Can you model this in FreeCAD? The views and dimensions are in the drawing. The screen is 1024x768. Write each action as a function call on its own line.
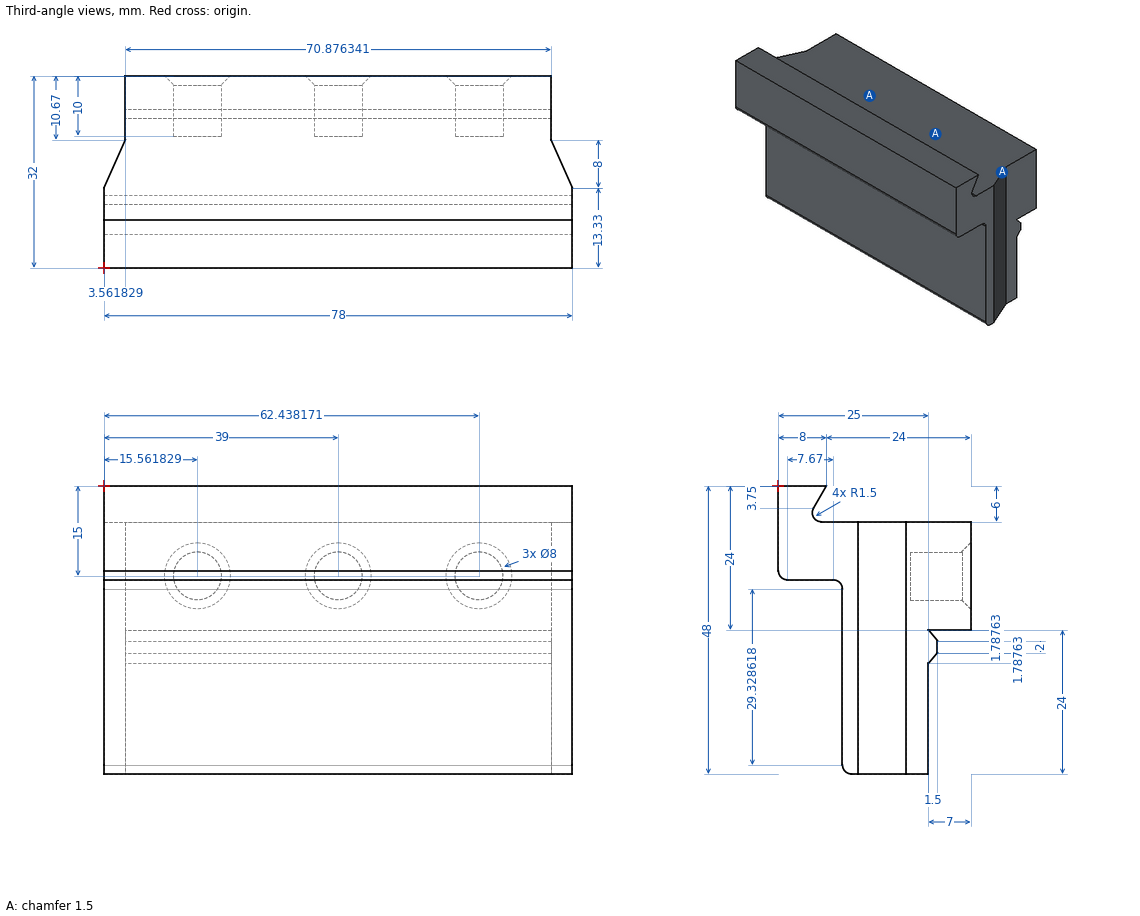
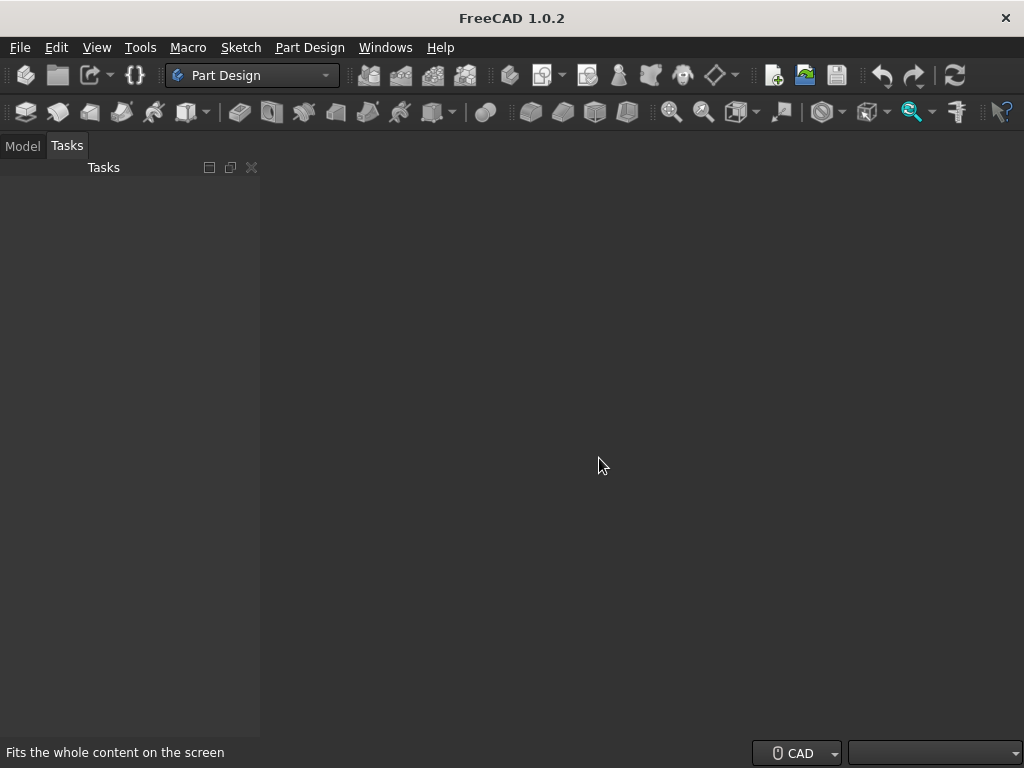
click(774, 76)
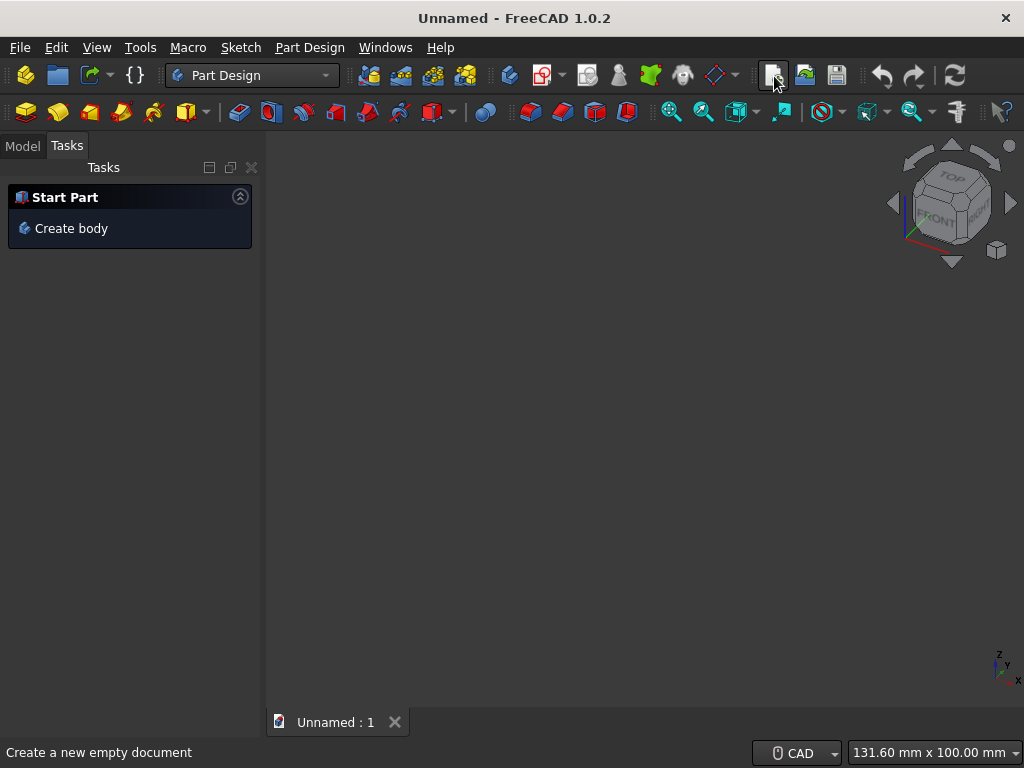
click(542, 76)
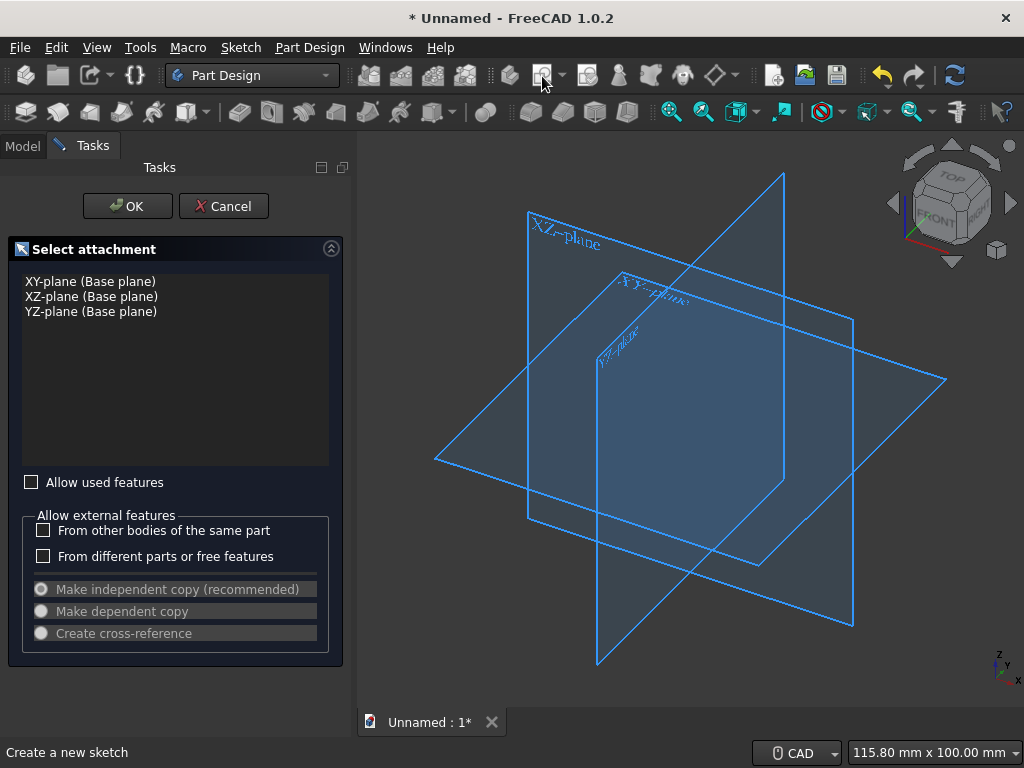
click(82, 282)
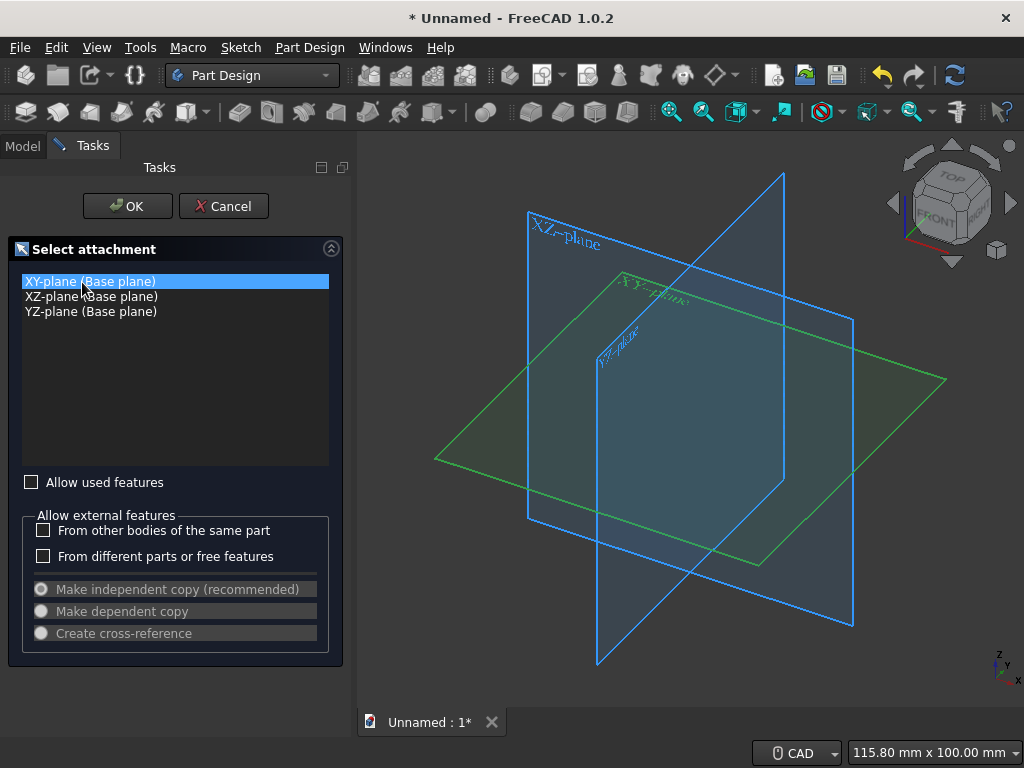
click(128, 206)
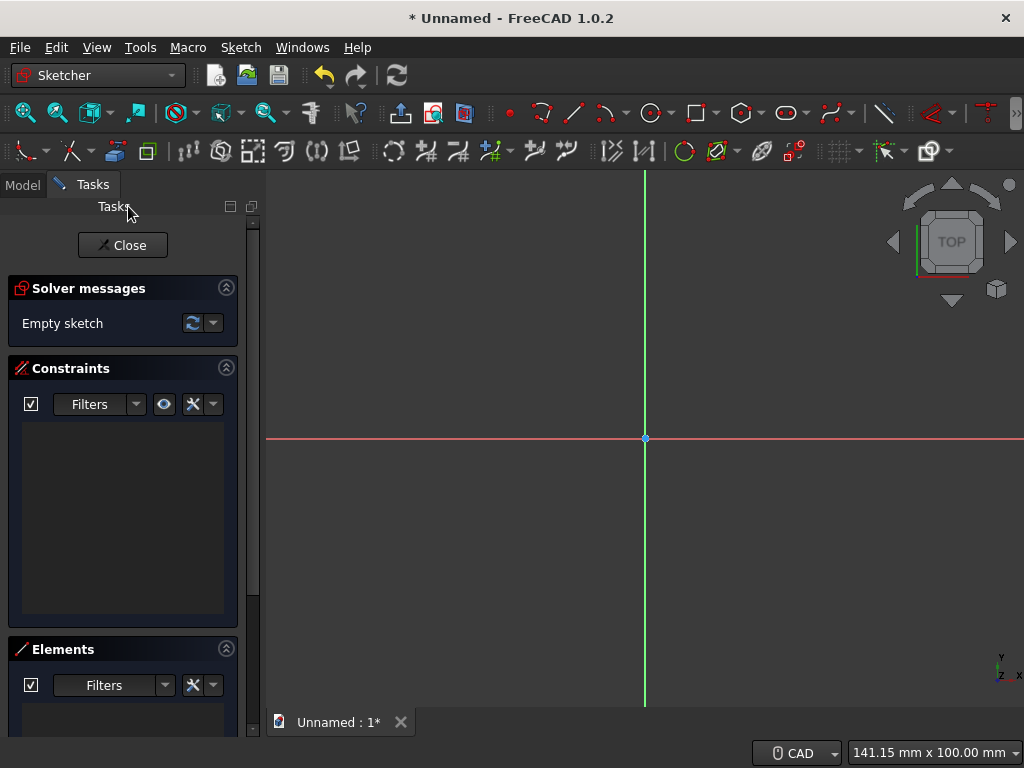
scroll(294, 613, down, 2)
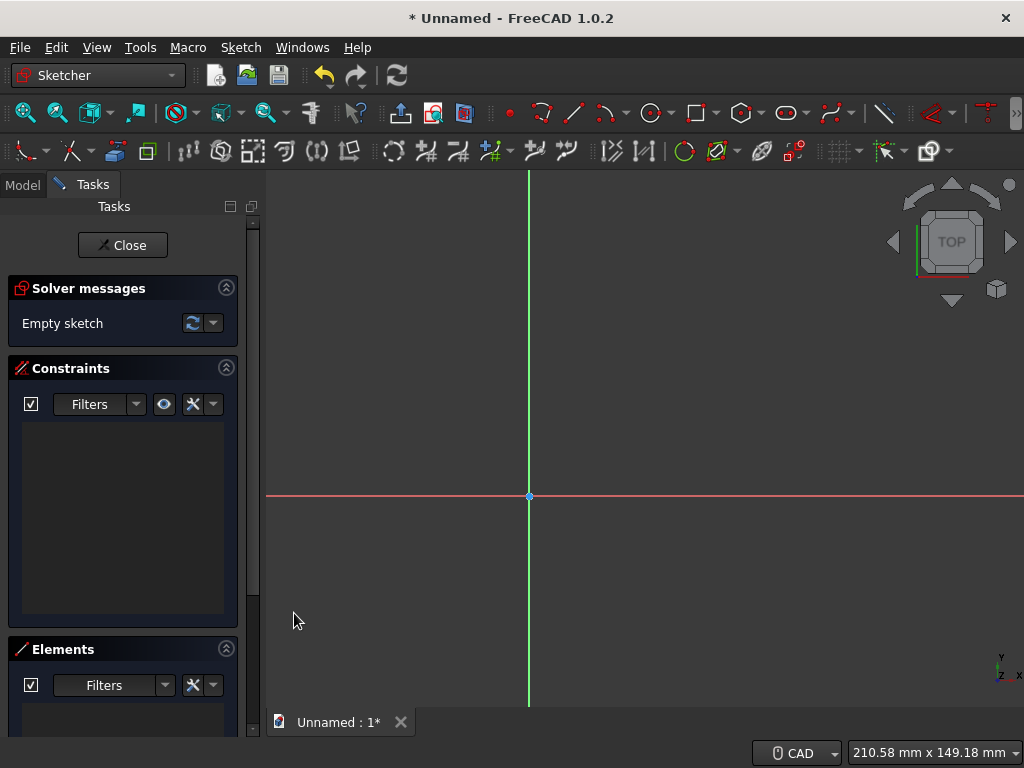
scroll(859, 439, up, 2)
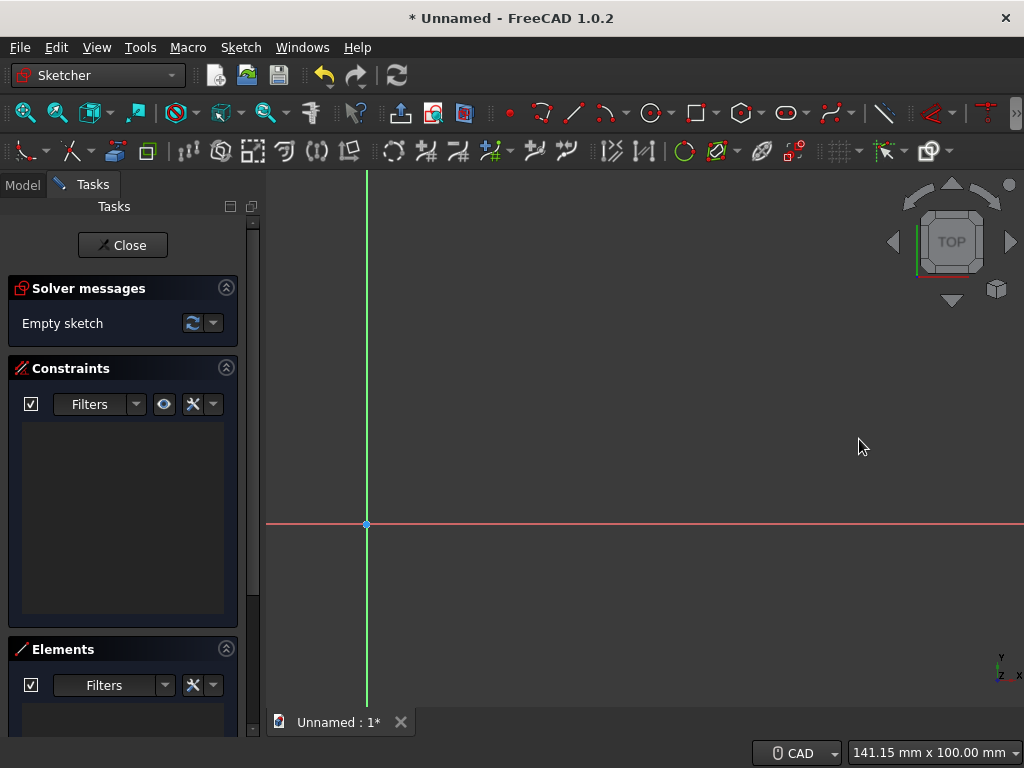
click(542, 114)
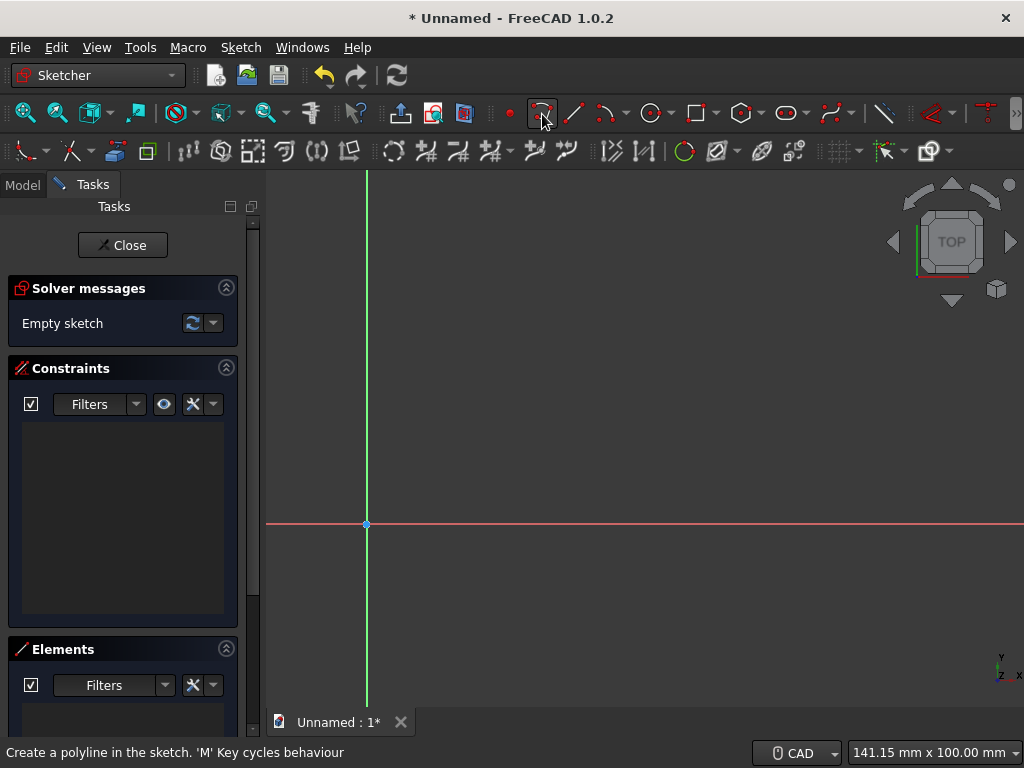
click(367, 524)
click(786, 515)
click(786, 453)
click(766, 410)
click(766, 352)
click(386, 352)
click(386, 410)
click(376, 453)
click(367, 524)
key(Escape)
key(Escape)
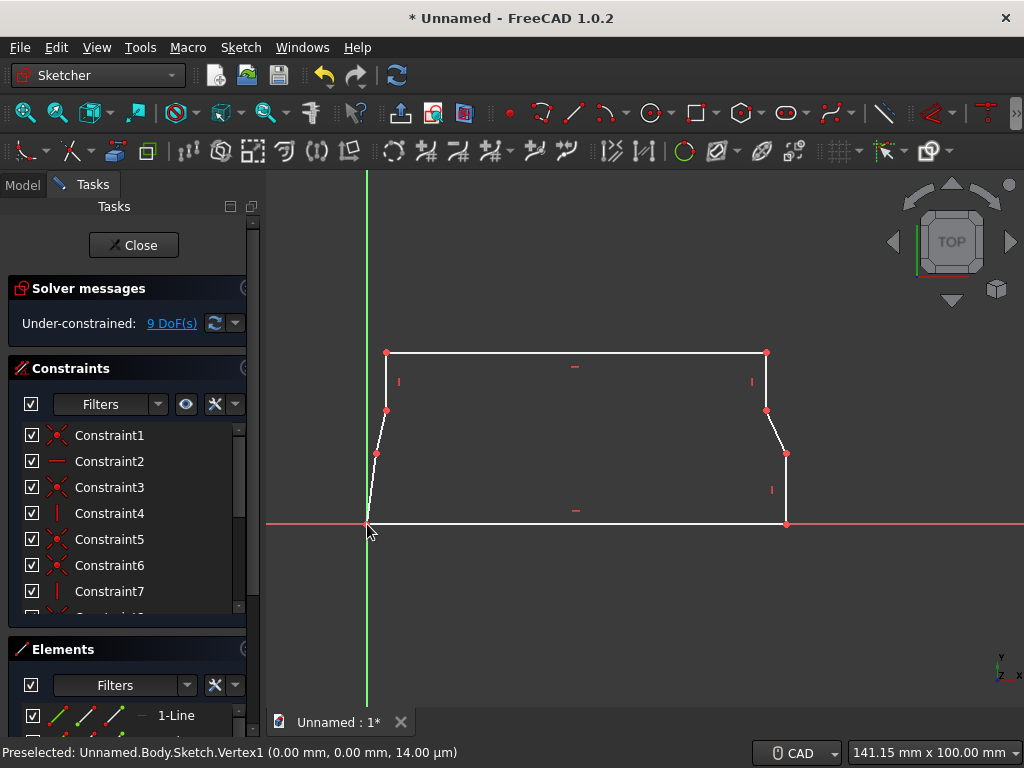
click(370, 503)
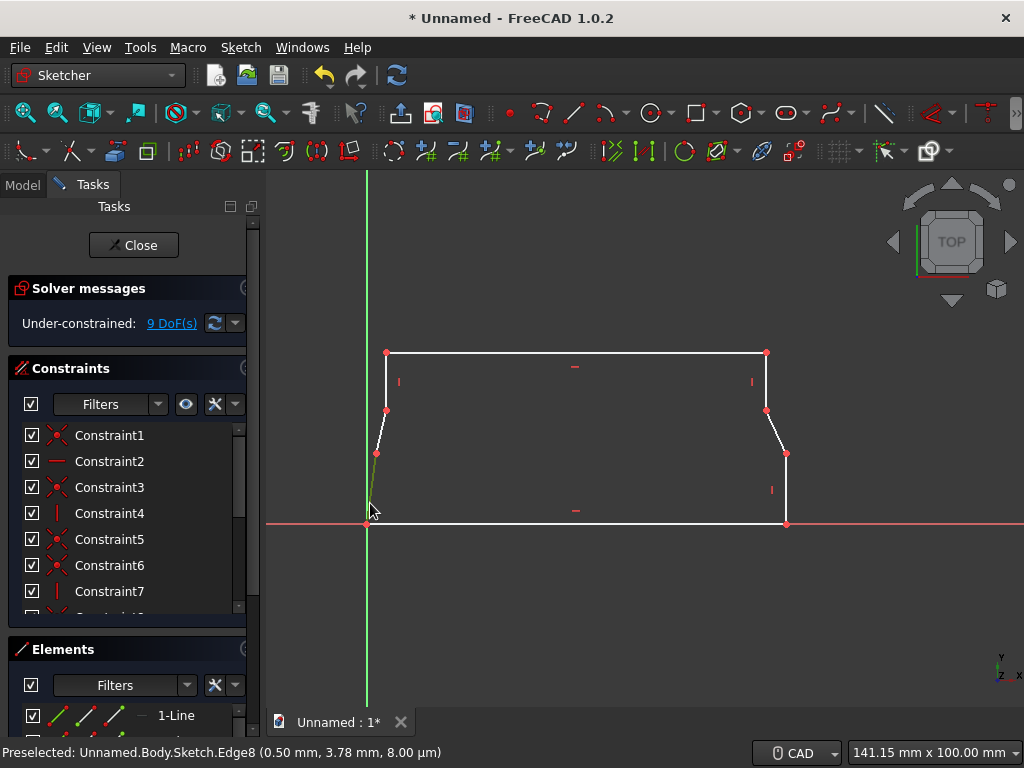
key(v)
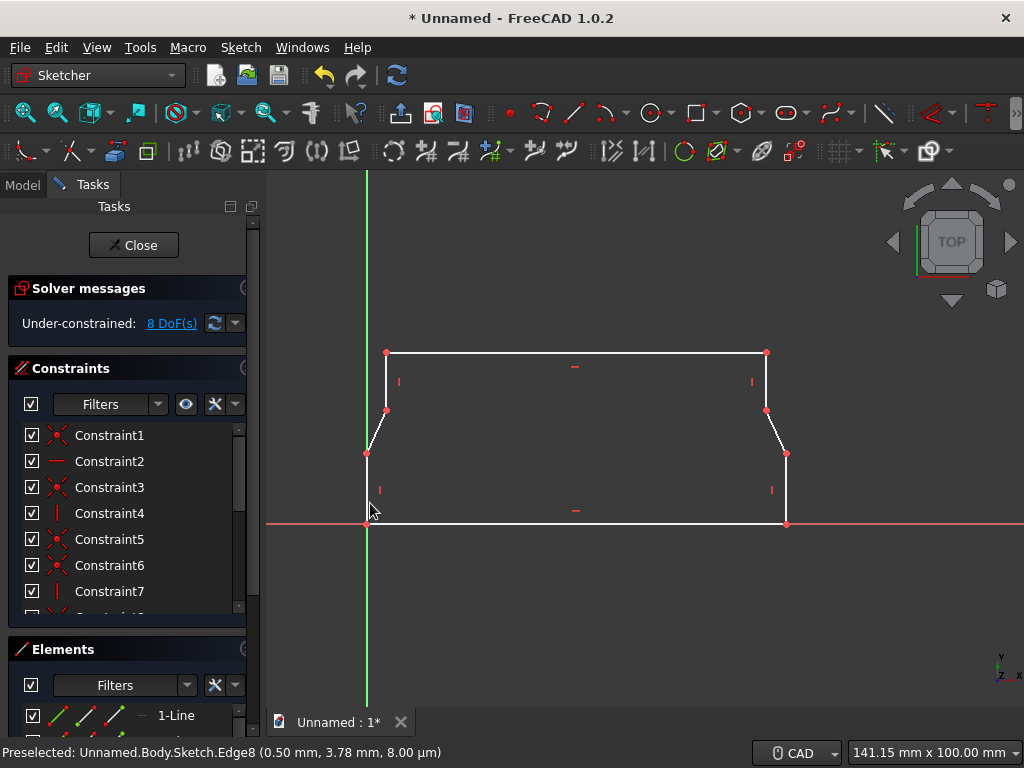
click(932, 114)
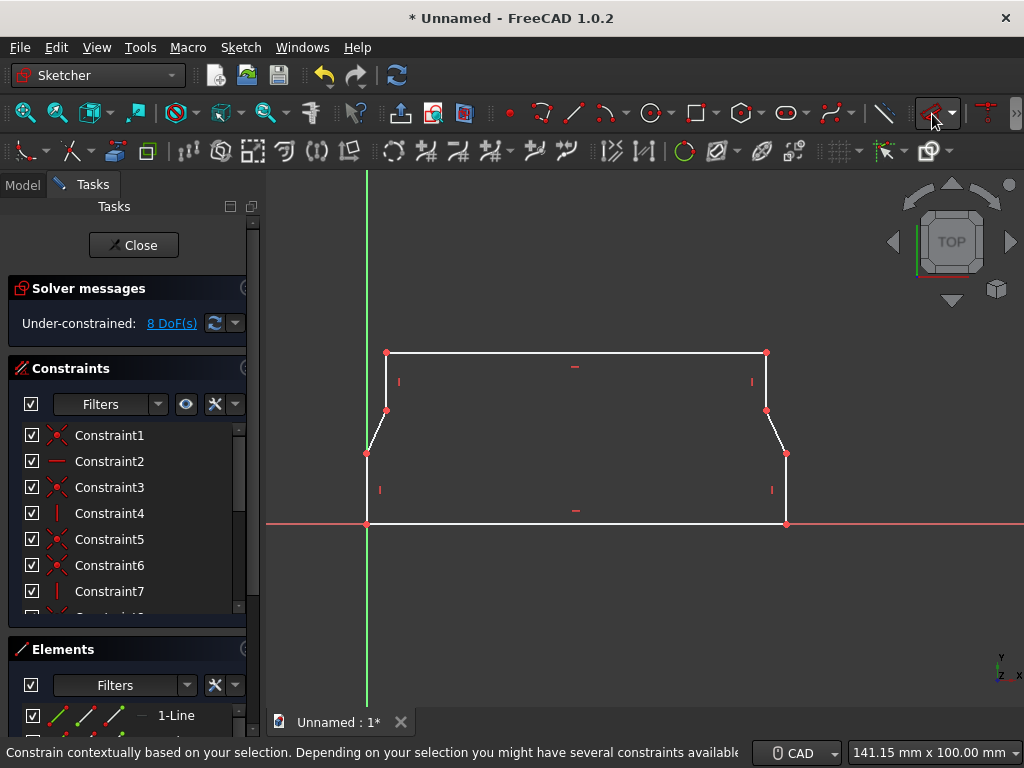
click(493, 524)
click(576, 558)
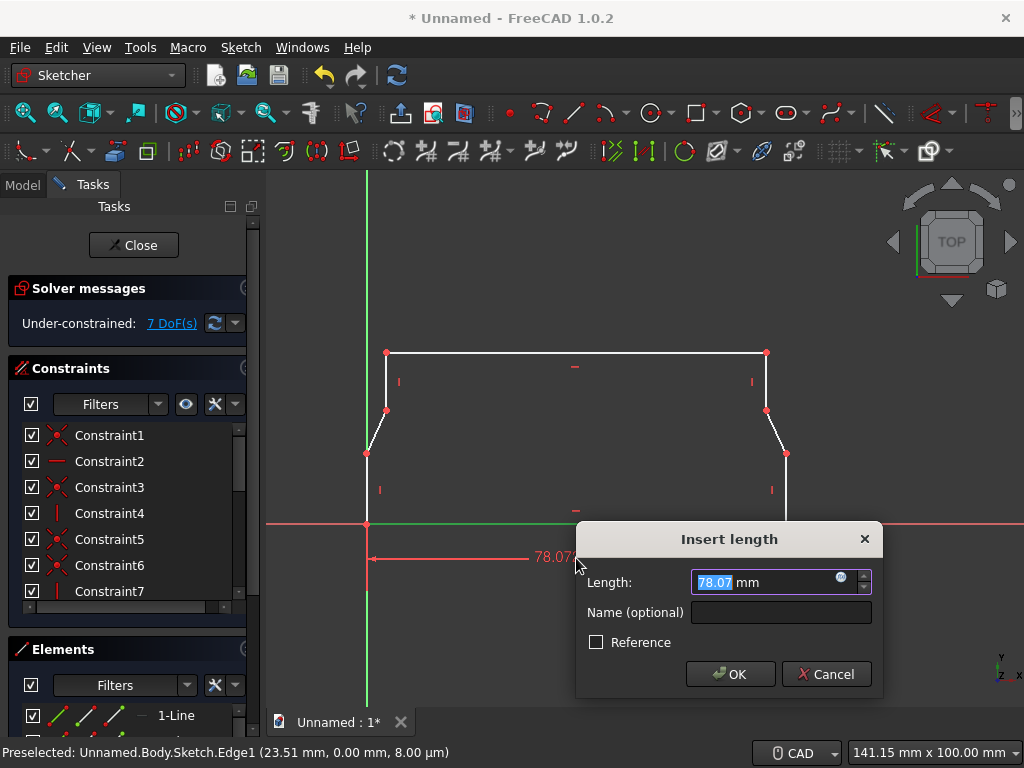
text(78)
key(Return)